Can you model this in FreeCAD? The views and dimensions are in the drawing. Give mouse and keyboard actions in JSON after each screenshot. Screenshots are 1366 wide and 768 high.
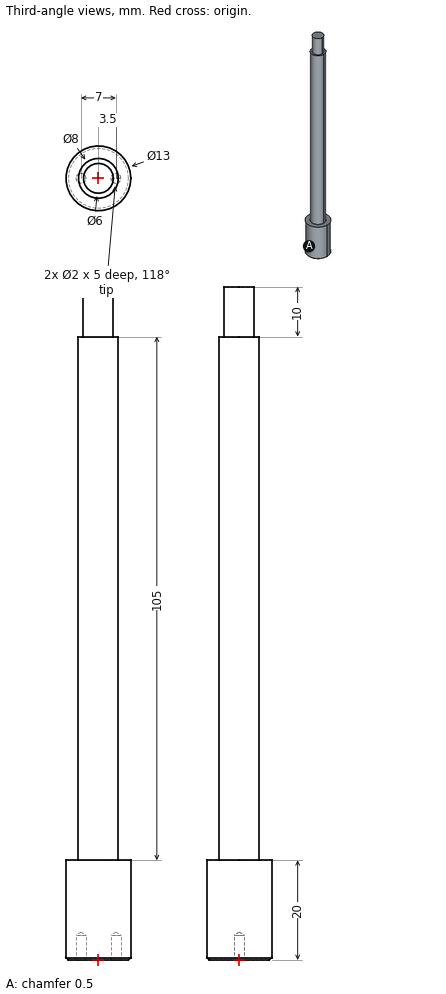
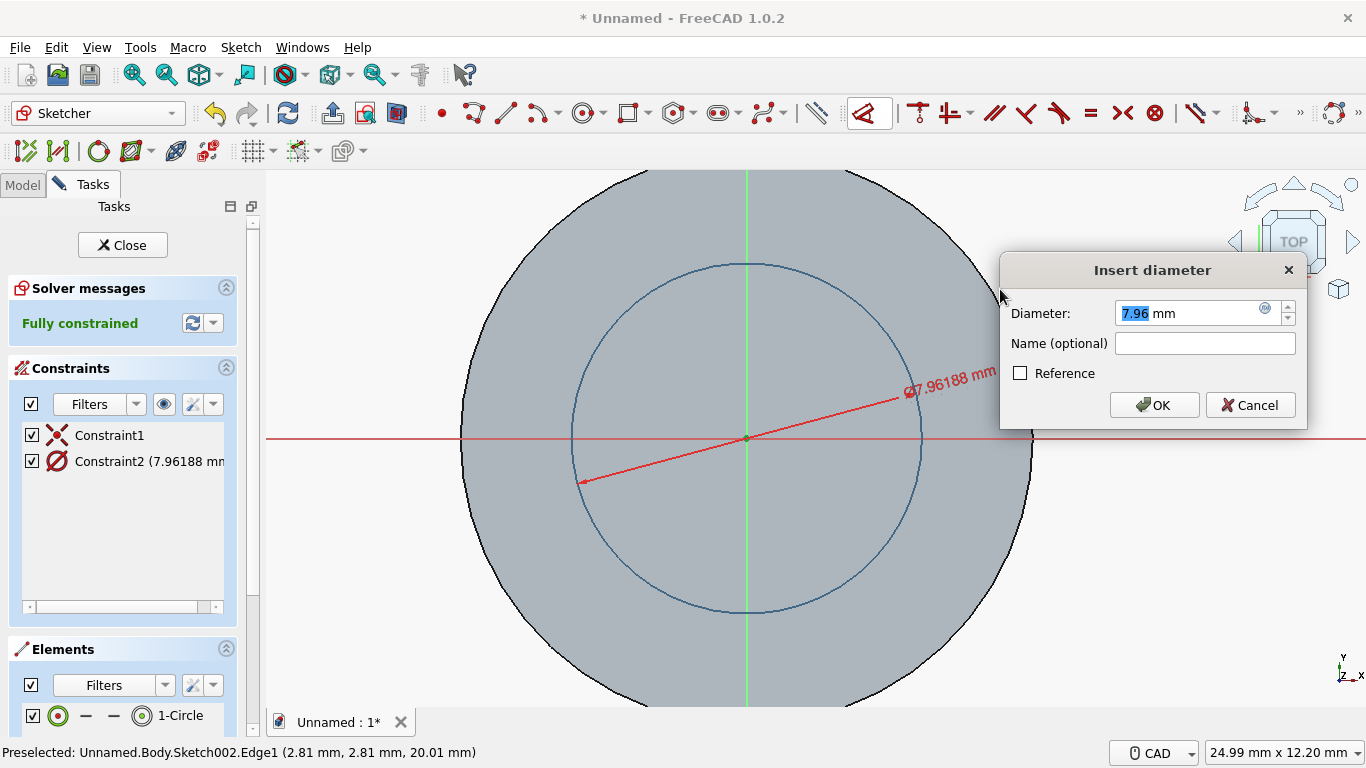
{"action": "type", "text": "8"}
{"action": "key", "text": "Return"}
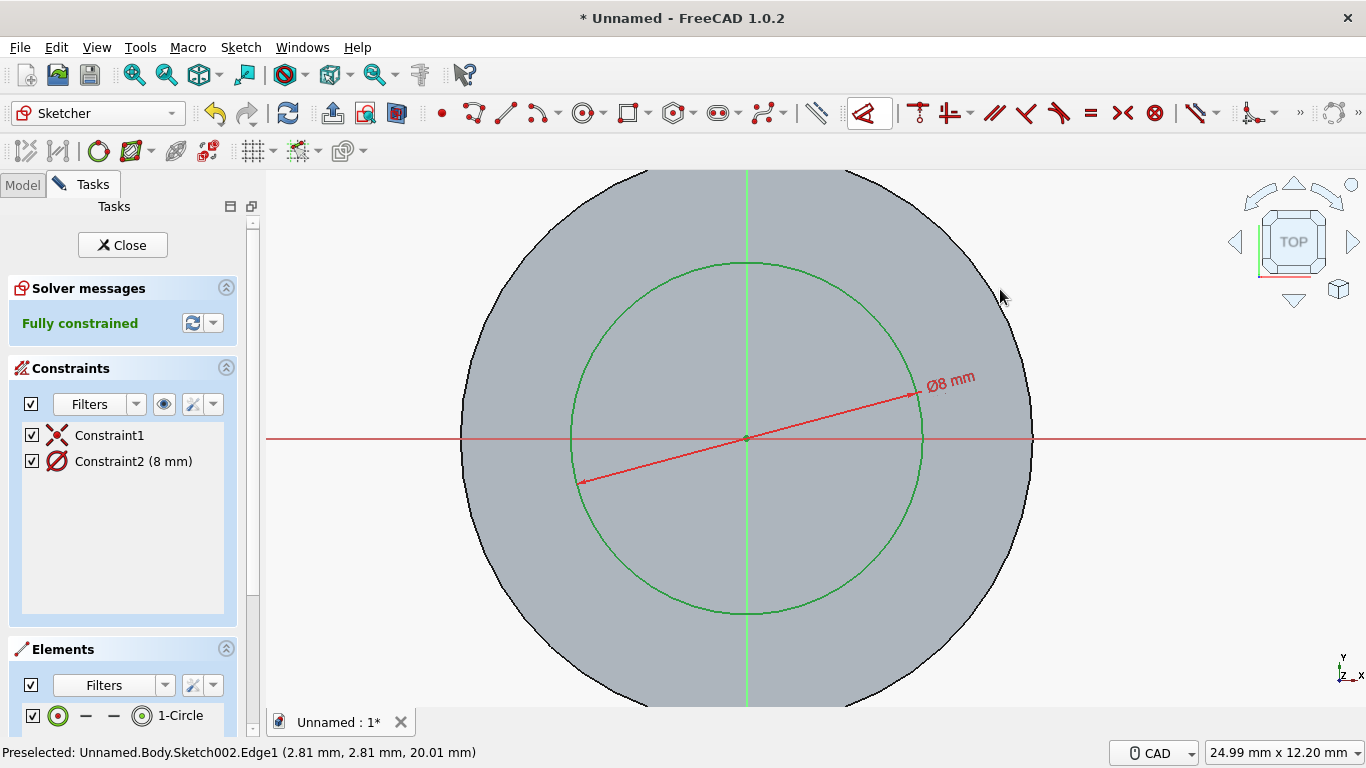
{"action": "left_click", "coordinate": [123, 245]}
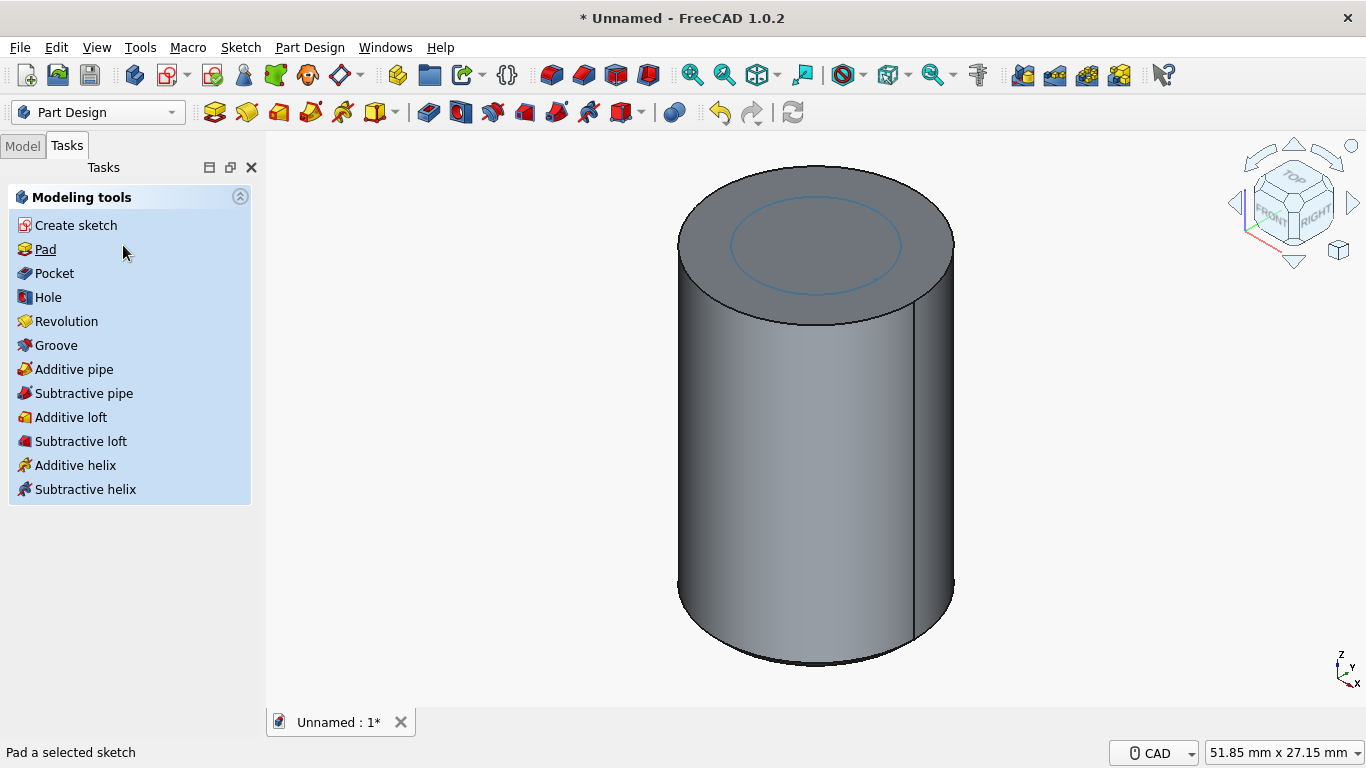
{"action": "left_click", "coordinate": [216, 112]}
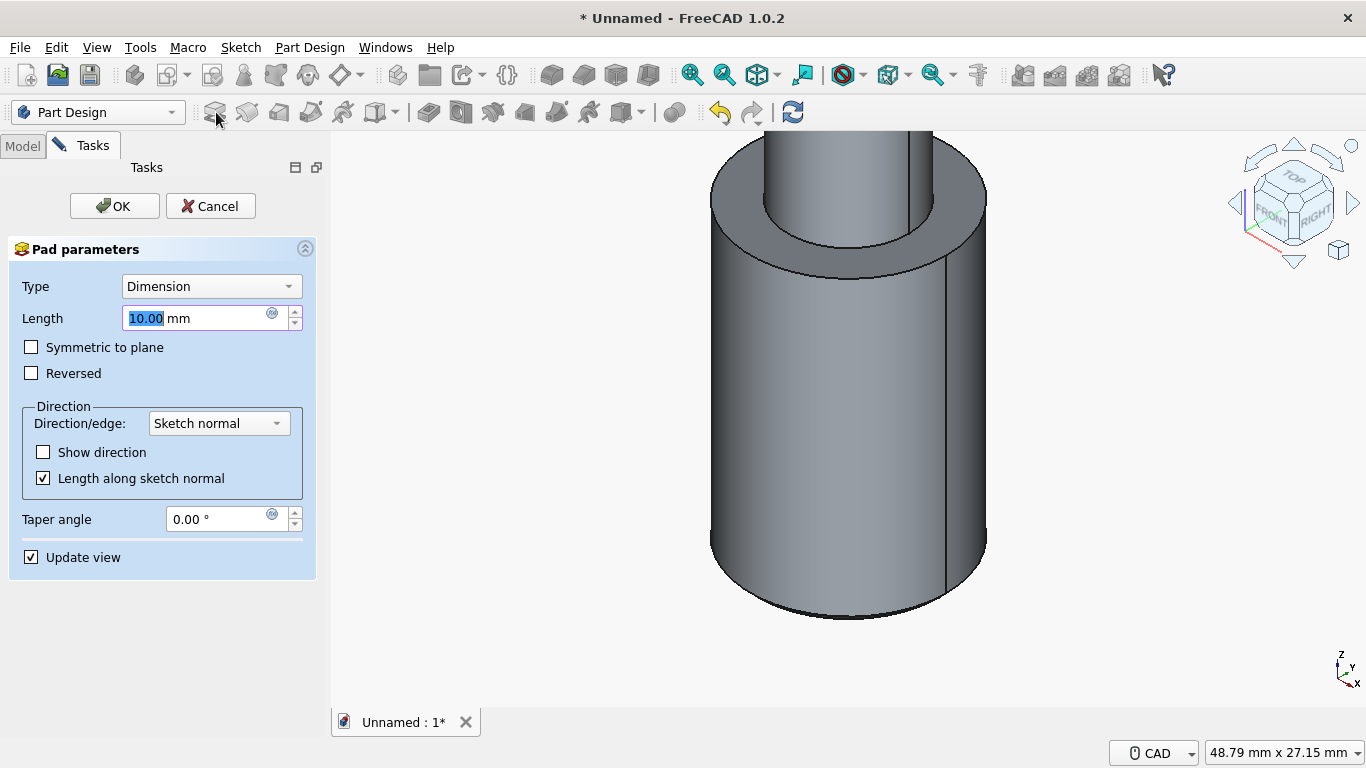
{"action": "type", "text": "105"}
{"action": "key", "text": "Tab"}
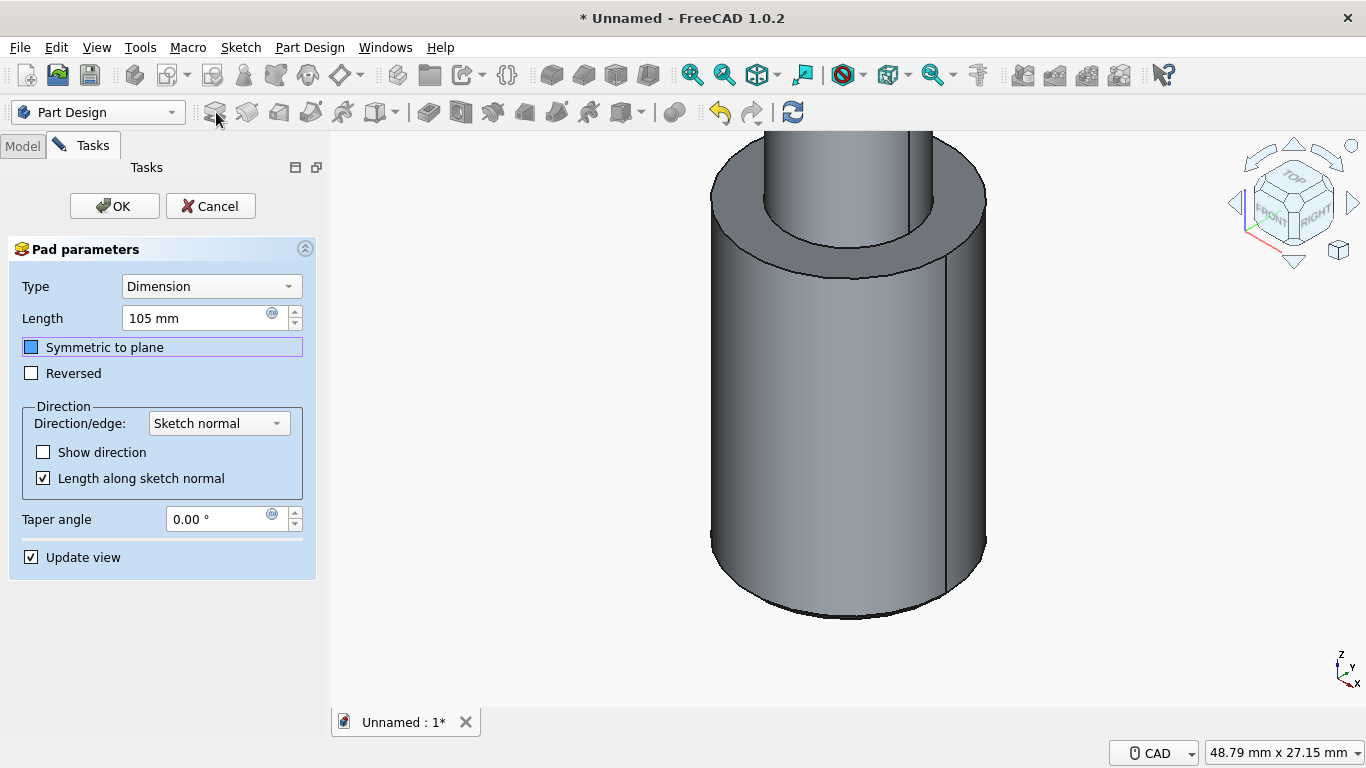
{"action": "left_click", "coordinate": [115, 206]}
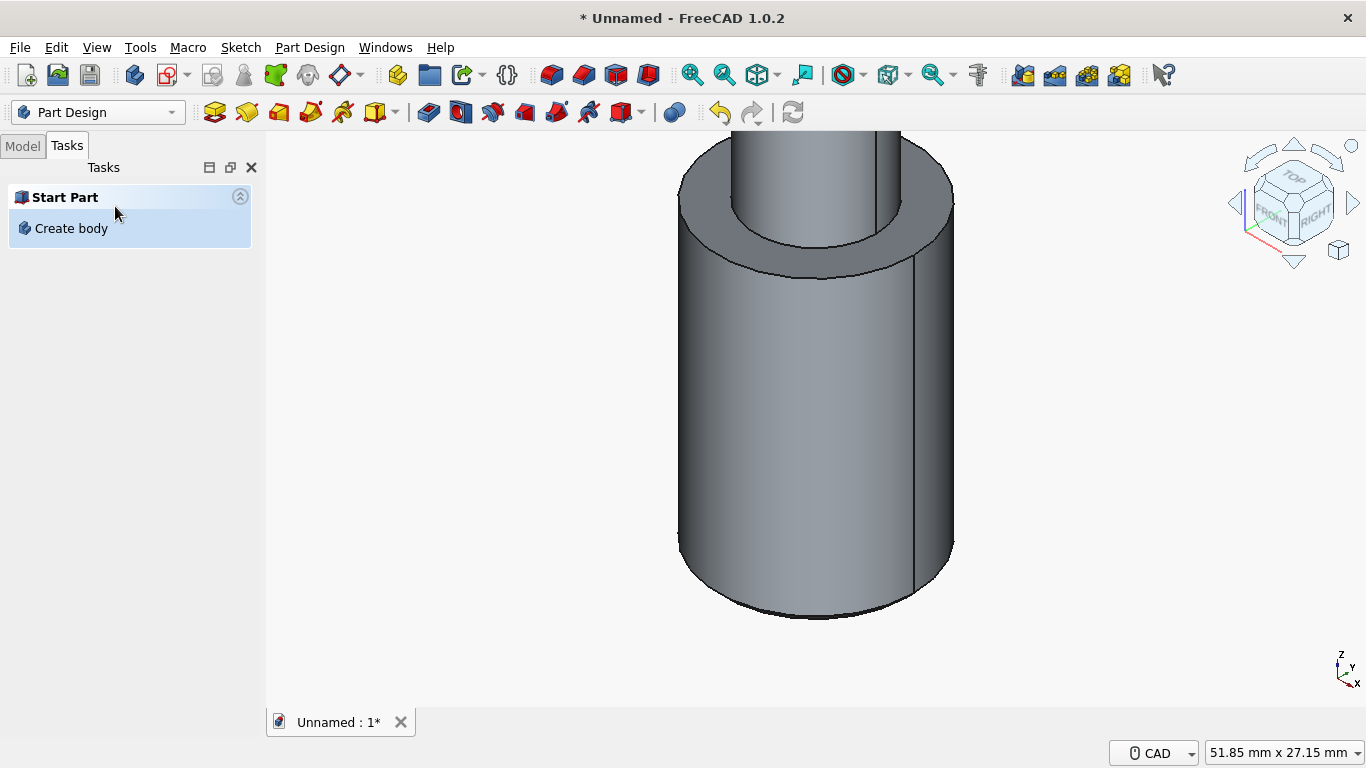
{"action": "key", "text": "v f"}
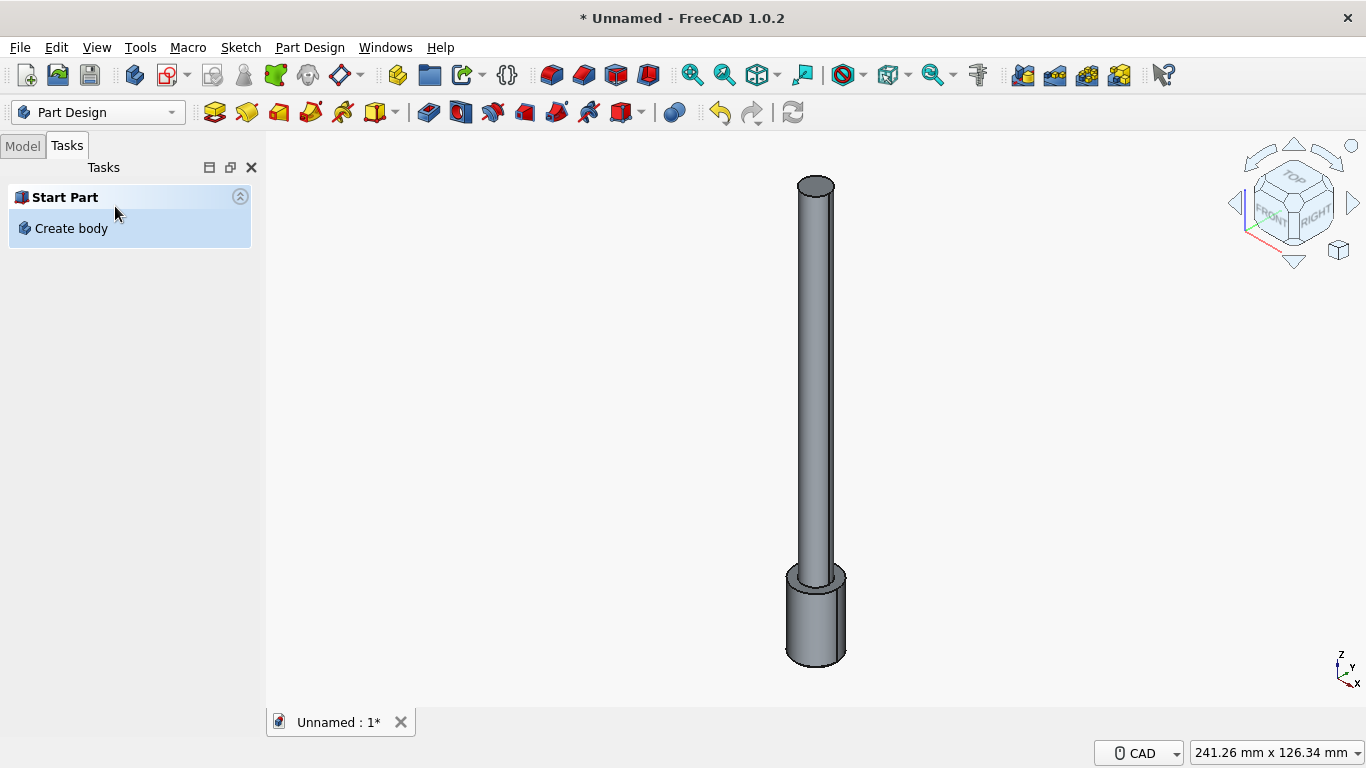
{"action": "left_click", "coordinate": [816, 185]}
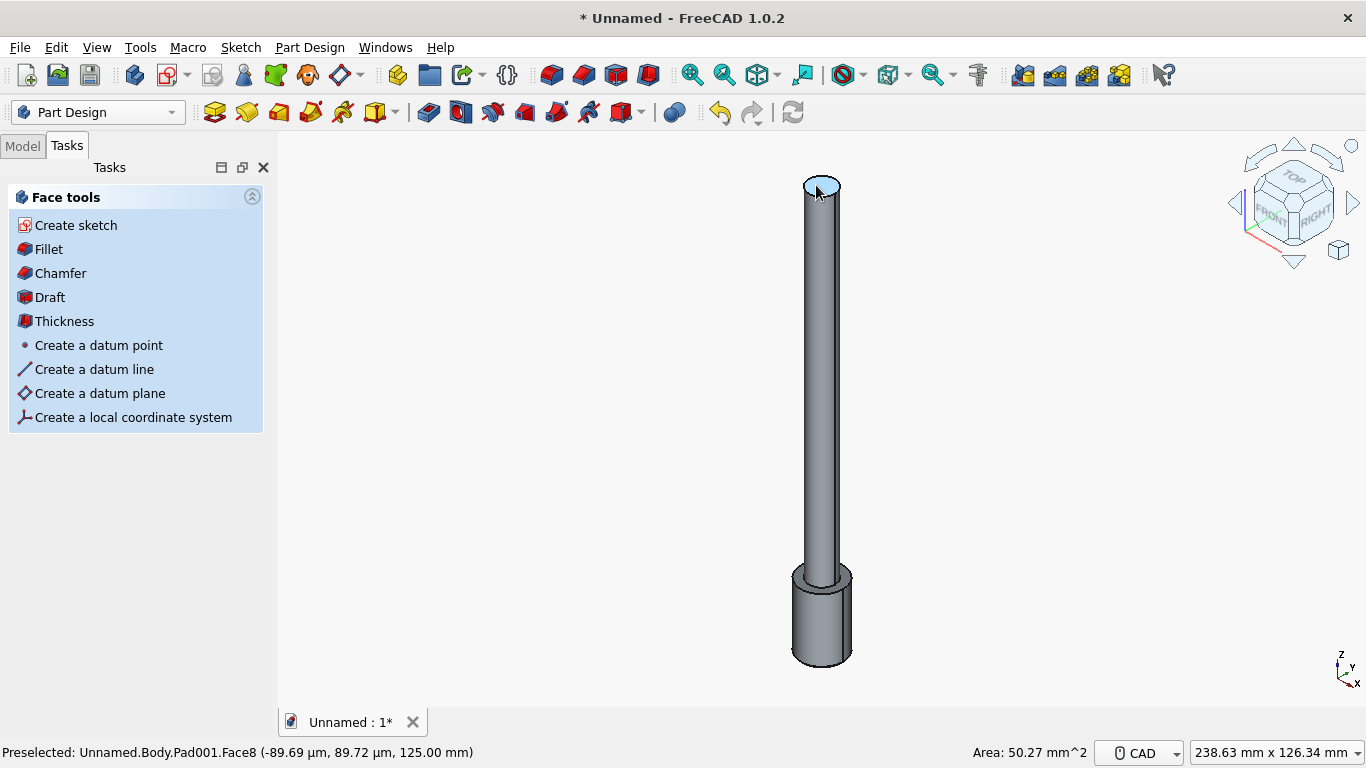
{"action": "left_click", "coordinate": [168, 76]}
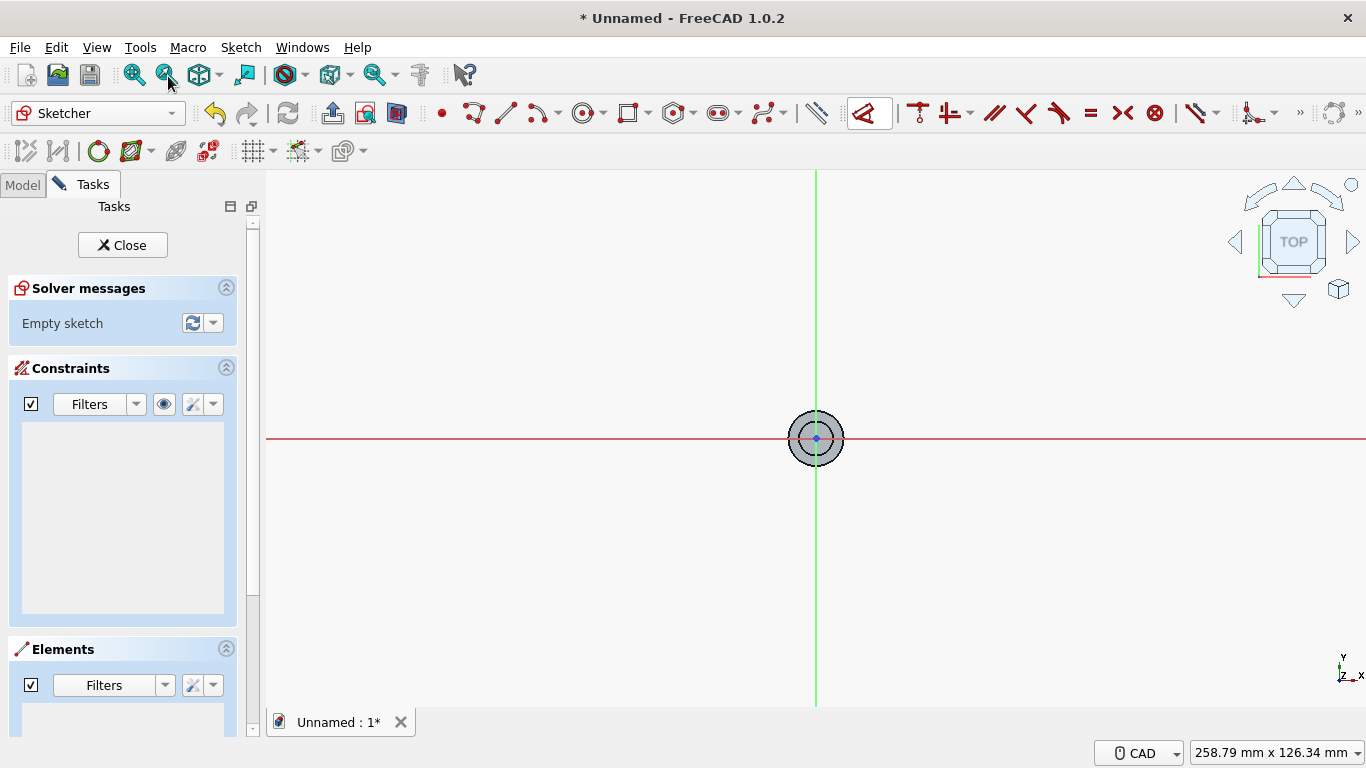
{"action": "scroll", "coordinate": [821, 438], "scroll_direction": "up", "scroll_amount": 13}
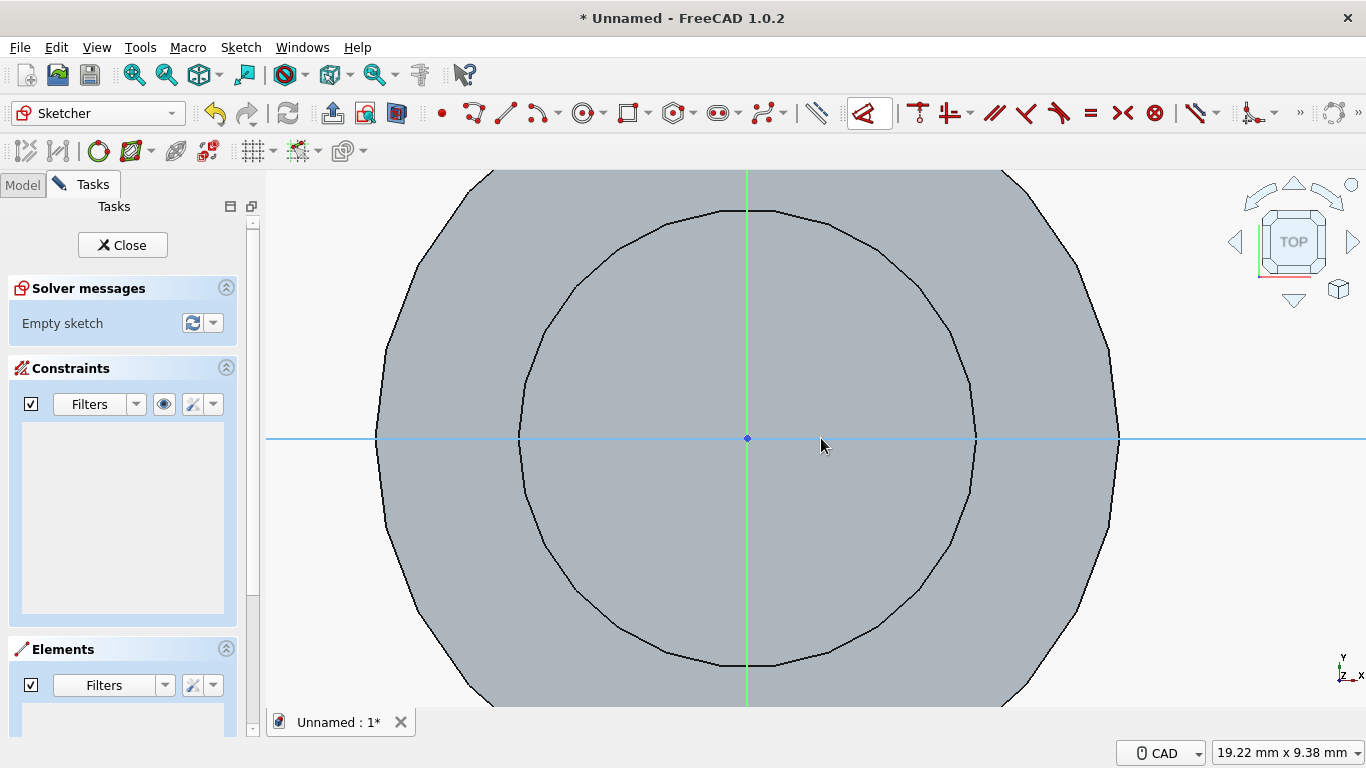
{"action": "left_click", "coordinate": [584, 114]}